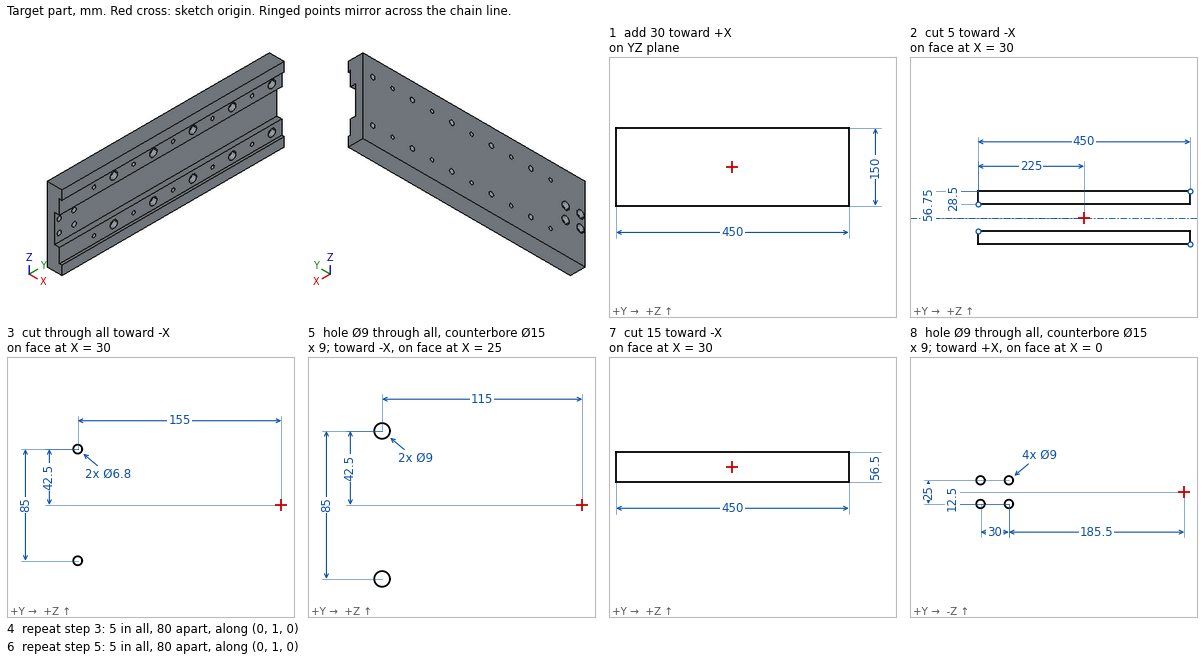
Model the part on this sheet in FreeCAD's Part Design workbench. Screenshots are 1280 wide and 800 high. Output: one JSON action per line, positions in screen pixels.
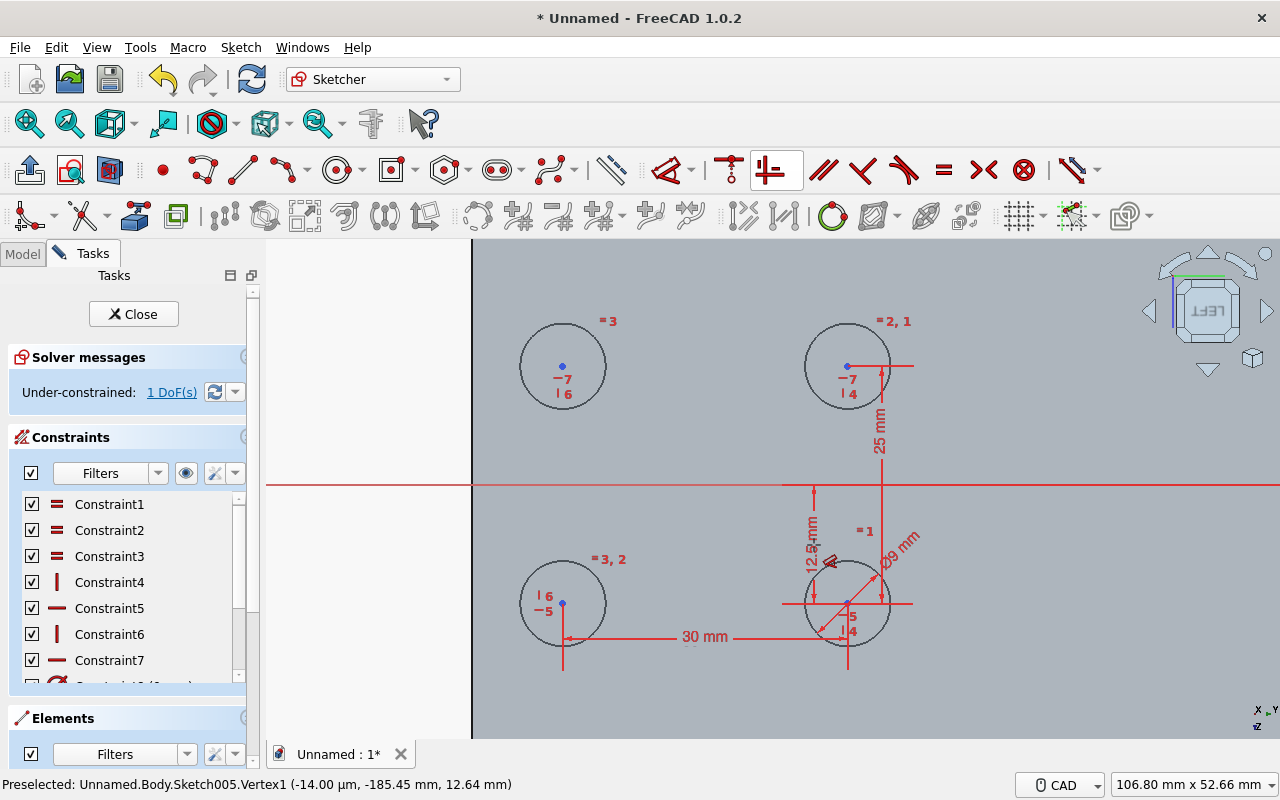
{"action": "left_click", "coordinate": [848, 604]}
{"action": "left_click", "coordinate": [981, 638]}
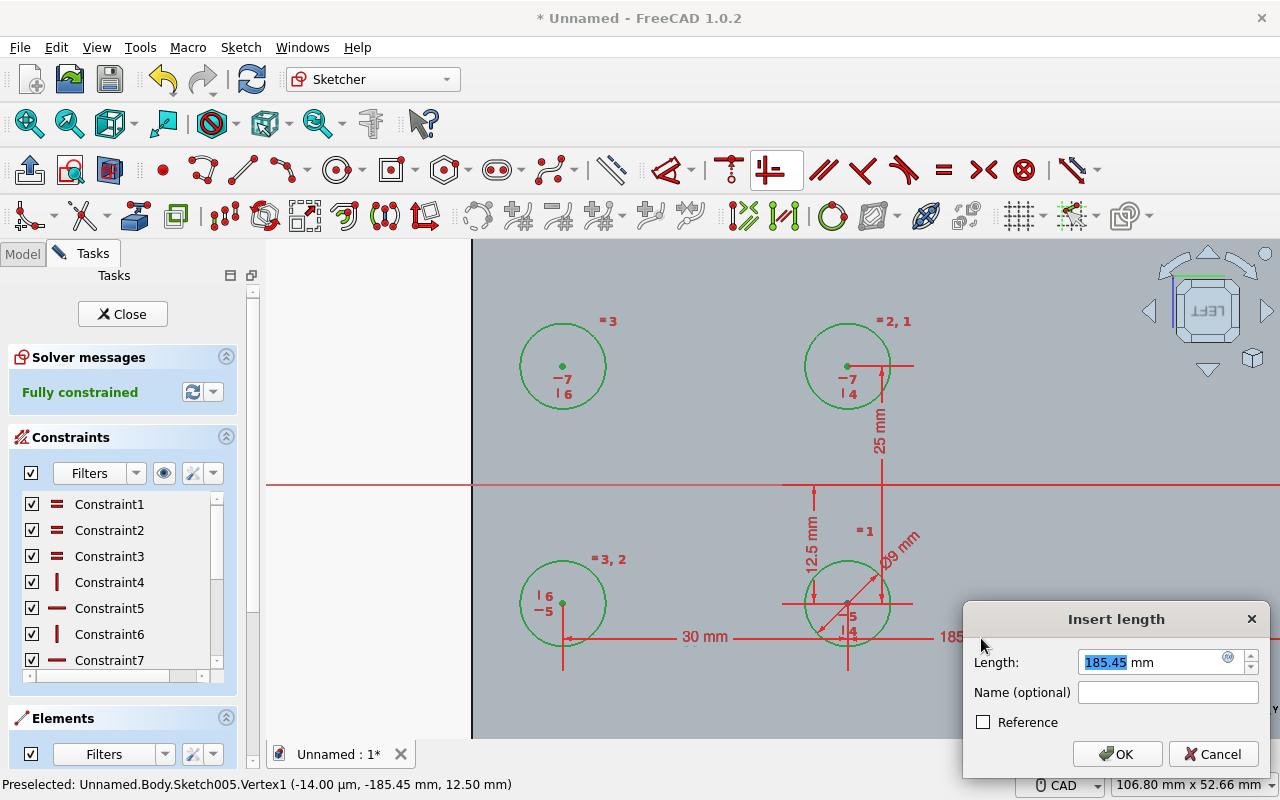
{"action": "type", "text": "185.5"}
{"action": "key", "text": "Return"}
{"action": "key", "text": "Escape"}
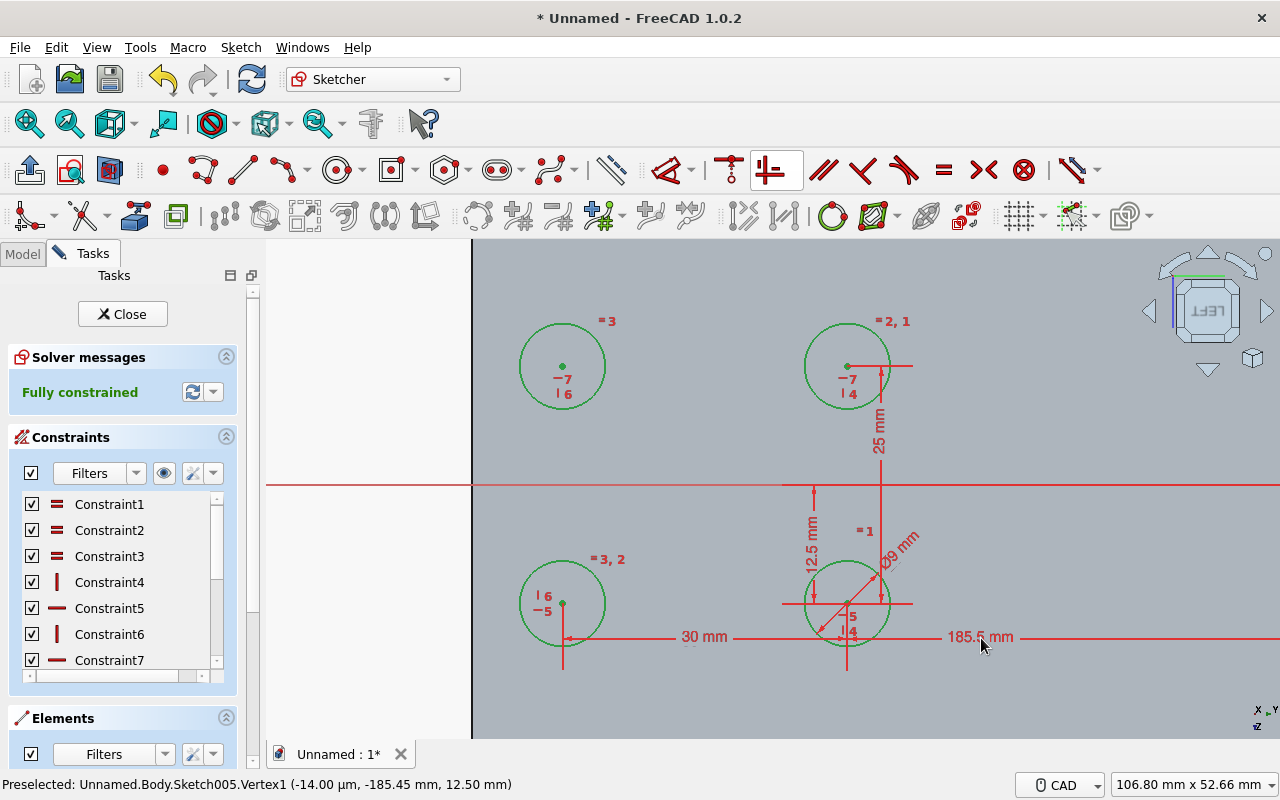
{"action": "left_click", "coordinate": [123, 314]}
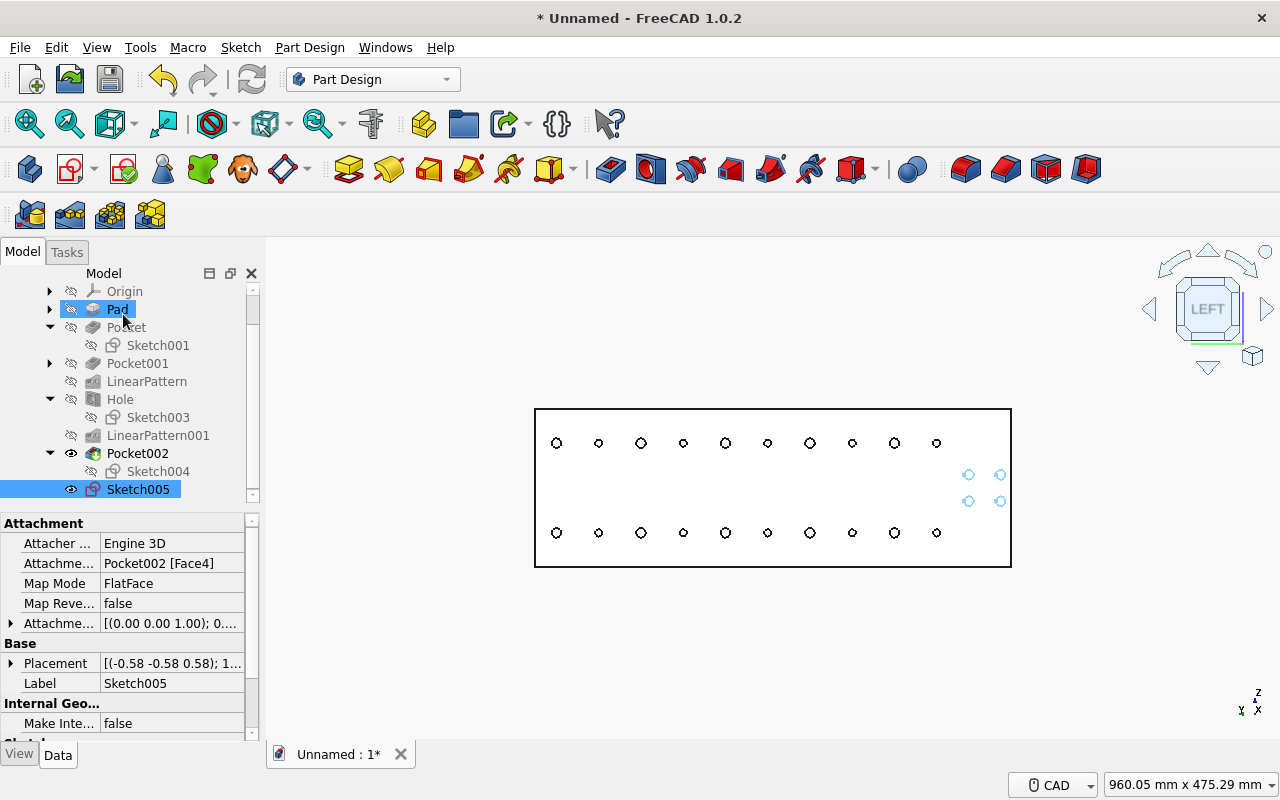
{"action": "left_click", "coordinate": [652, 170]}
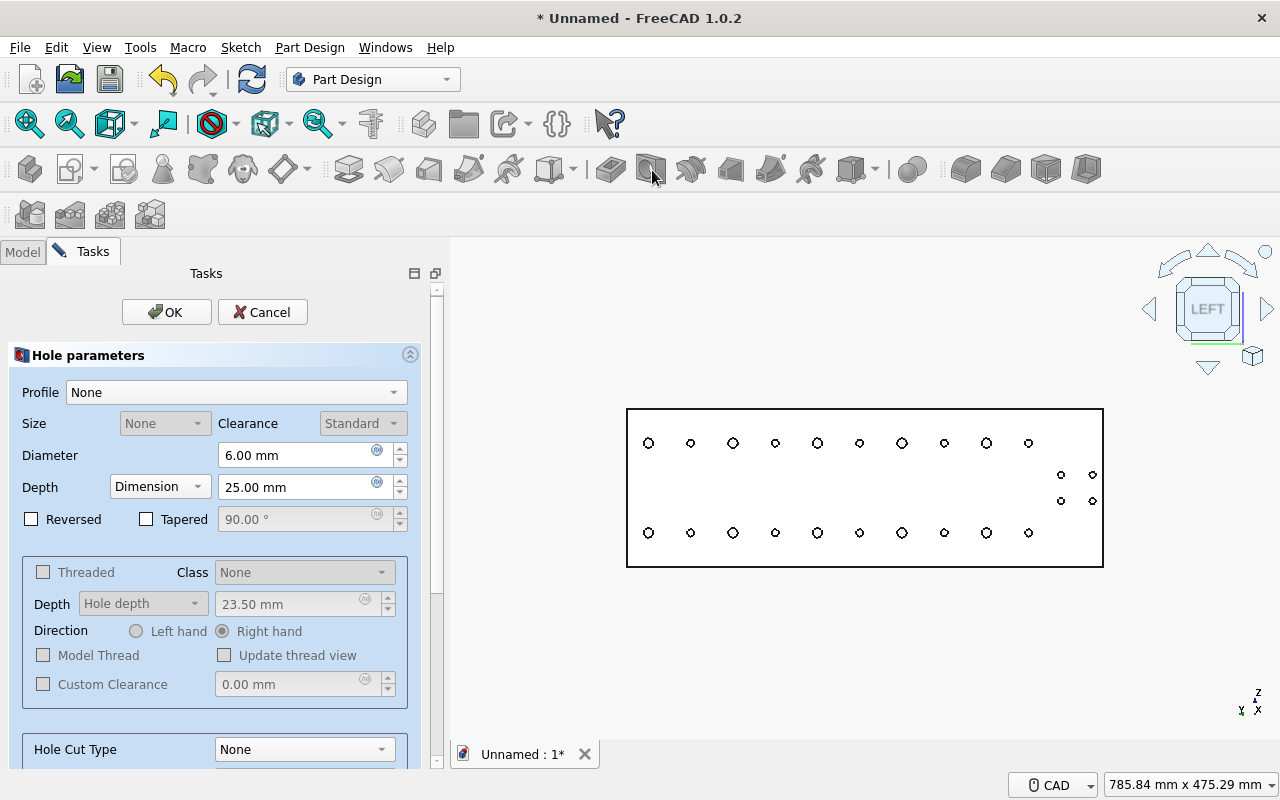
{"action": "triple_click", "coordinate": [305, 455]}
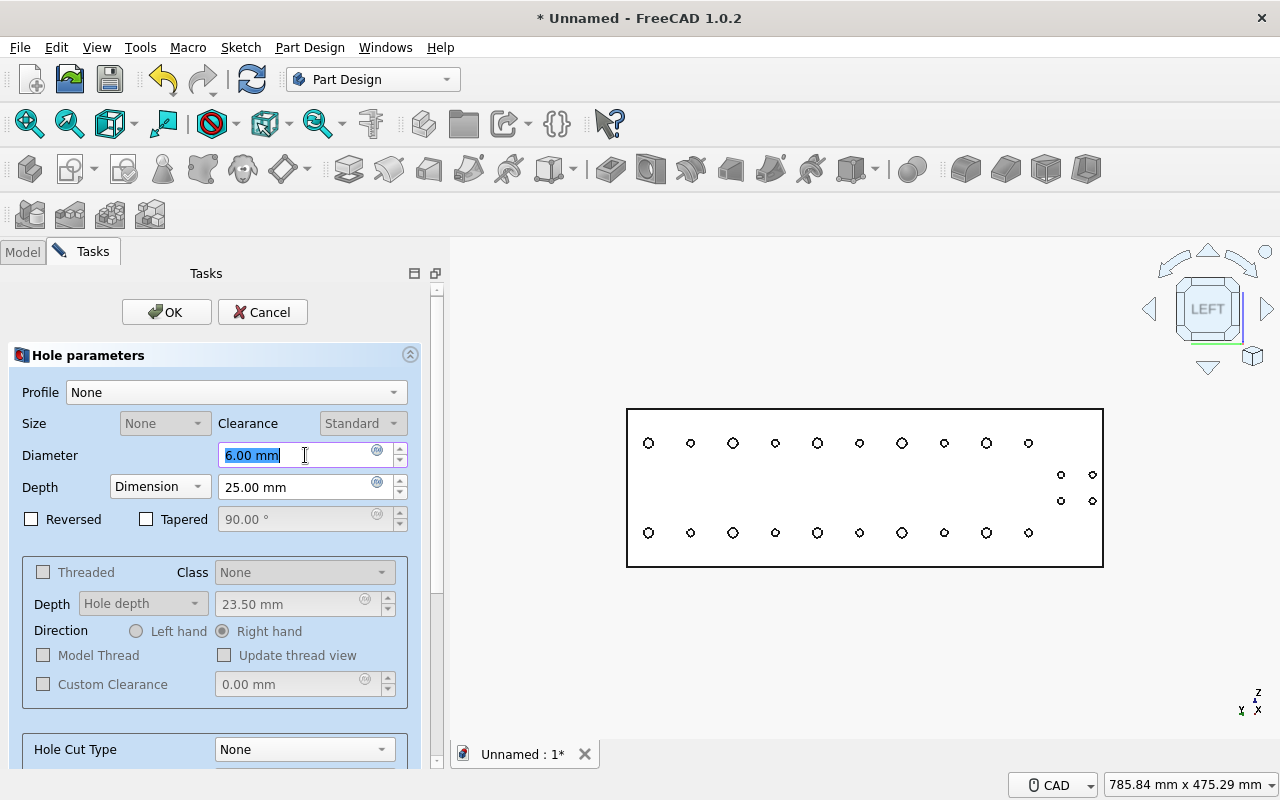
{"action": "type", "text": "9"}
{"action": "key", "text": "Tab"}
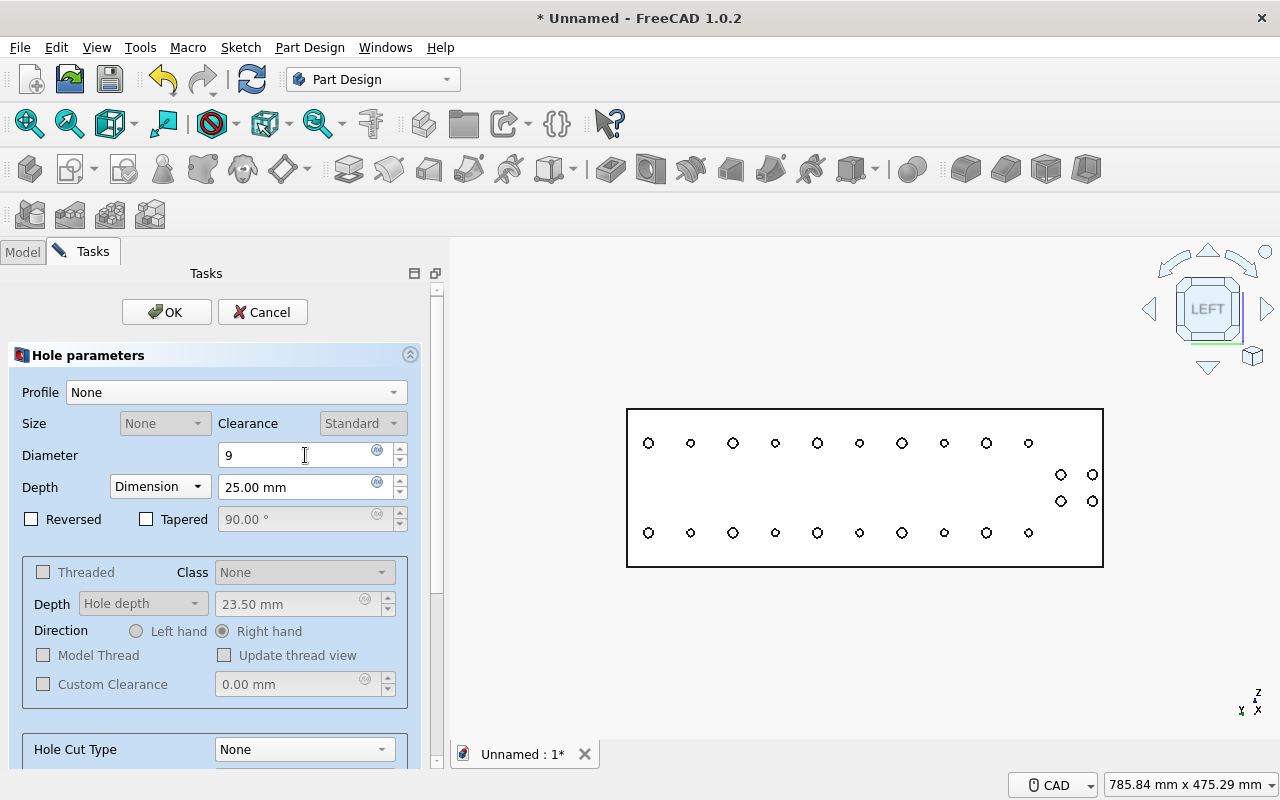
{"action": "left_click", "coordinate": [161, 486]}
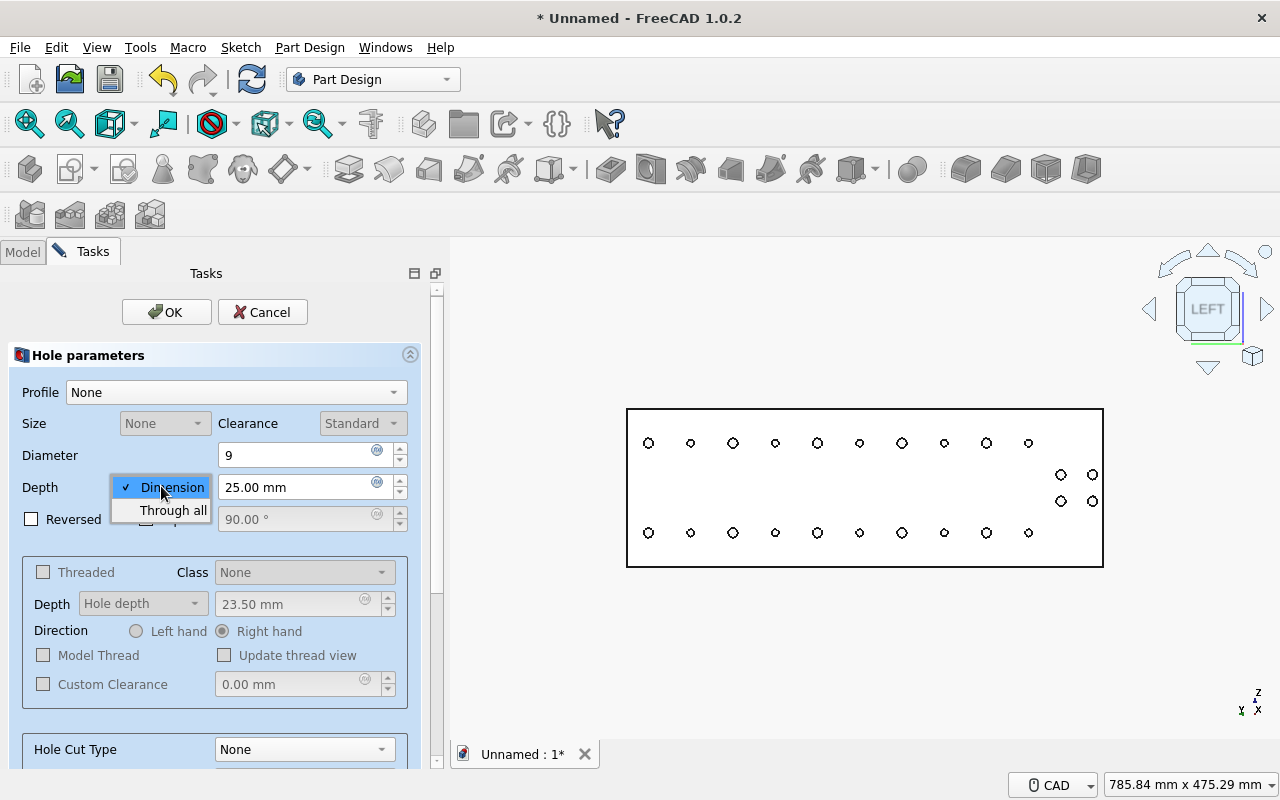
{"action": "left_click", "coordinate": [160, 510]}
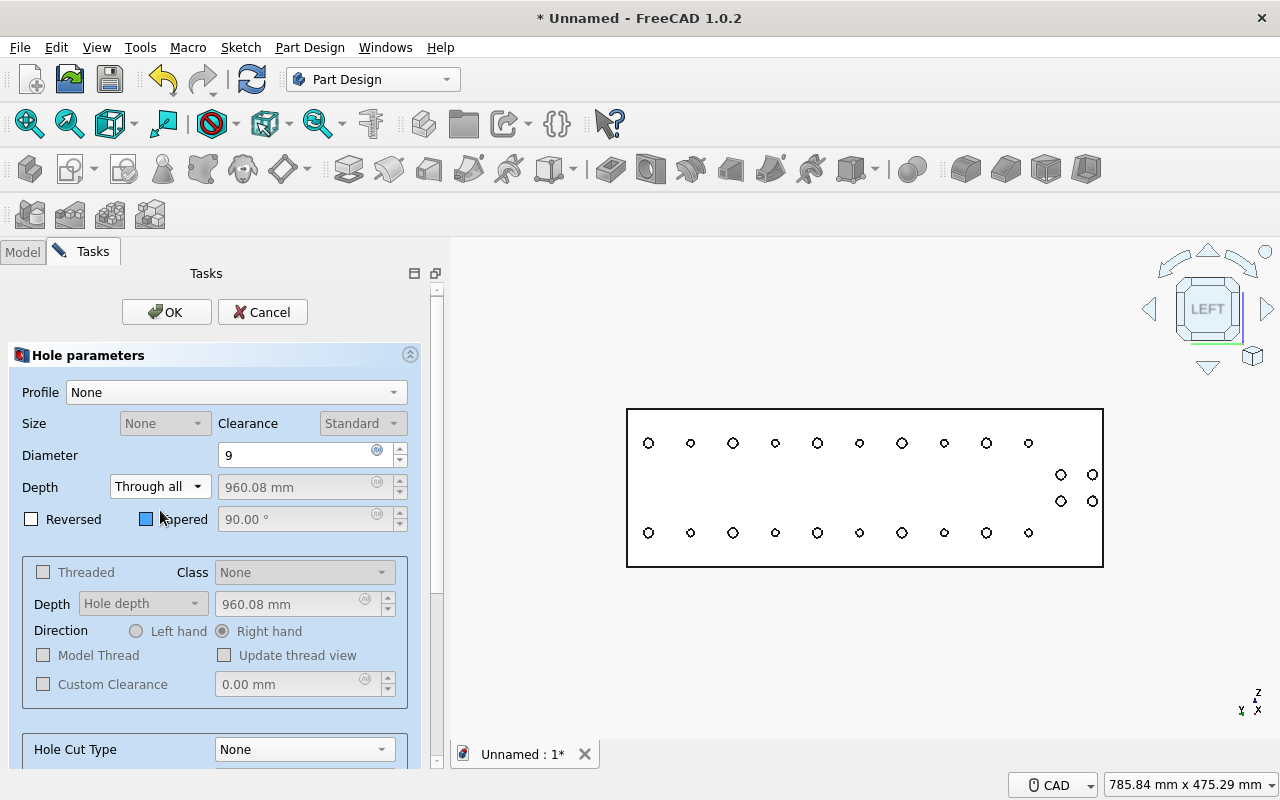
{"action": "left_click", "coordinate": [306, 750]}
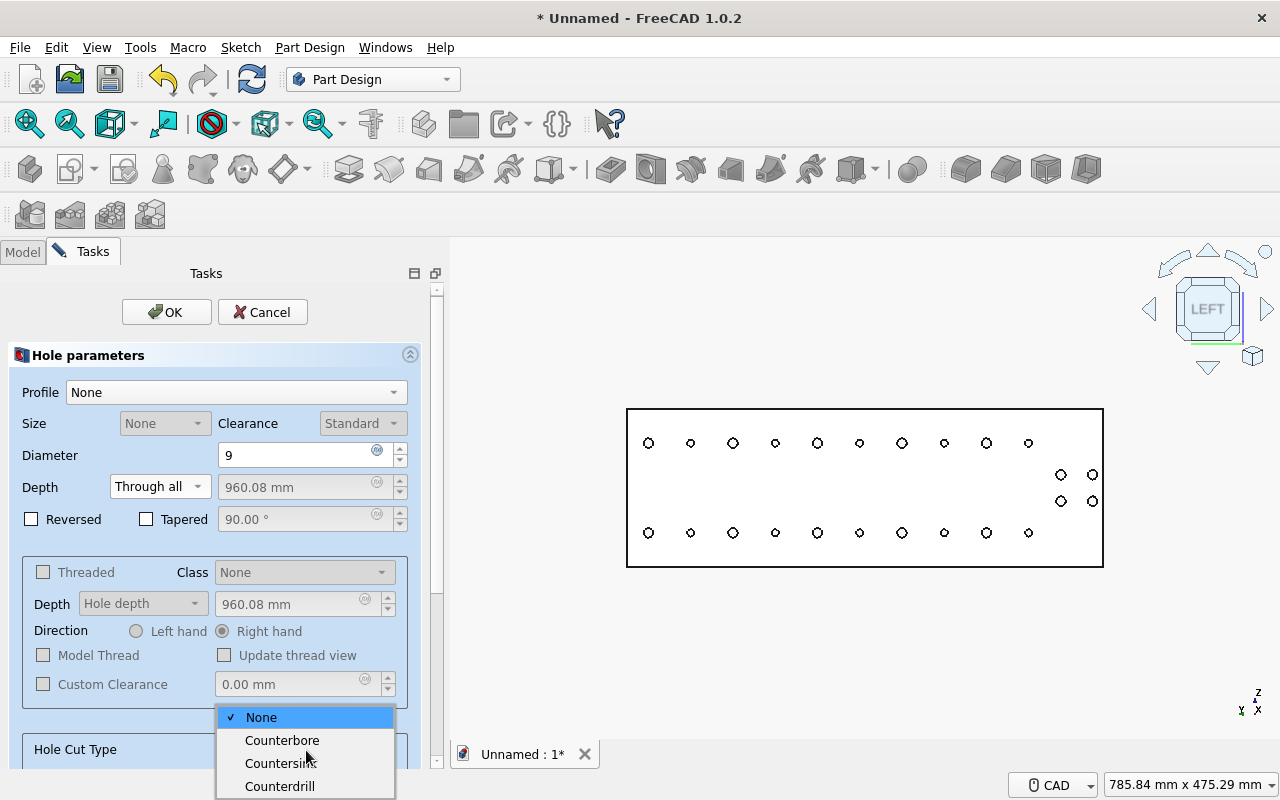
{"action": "left_click", "coordinate": [304, 740]}